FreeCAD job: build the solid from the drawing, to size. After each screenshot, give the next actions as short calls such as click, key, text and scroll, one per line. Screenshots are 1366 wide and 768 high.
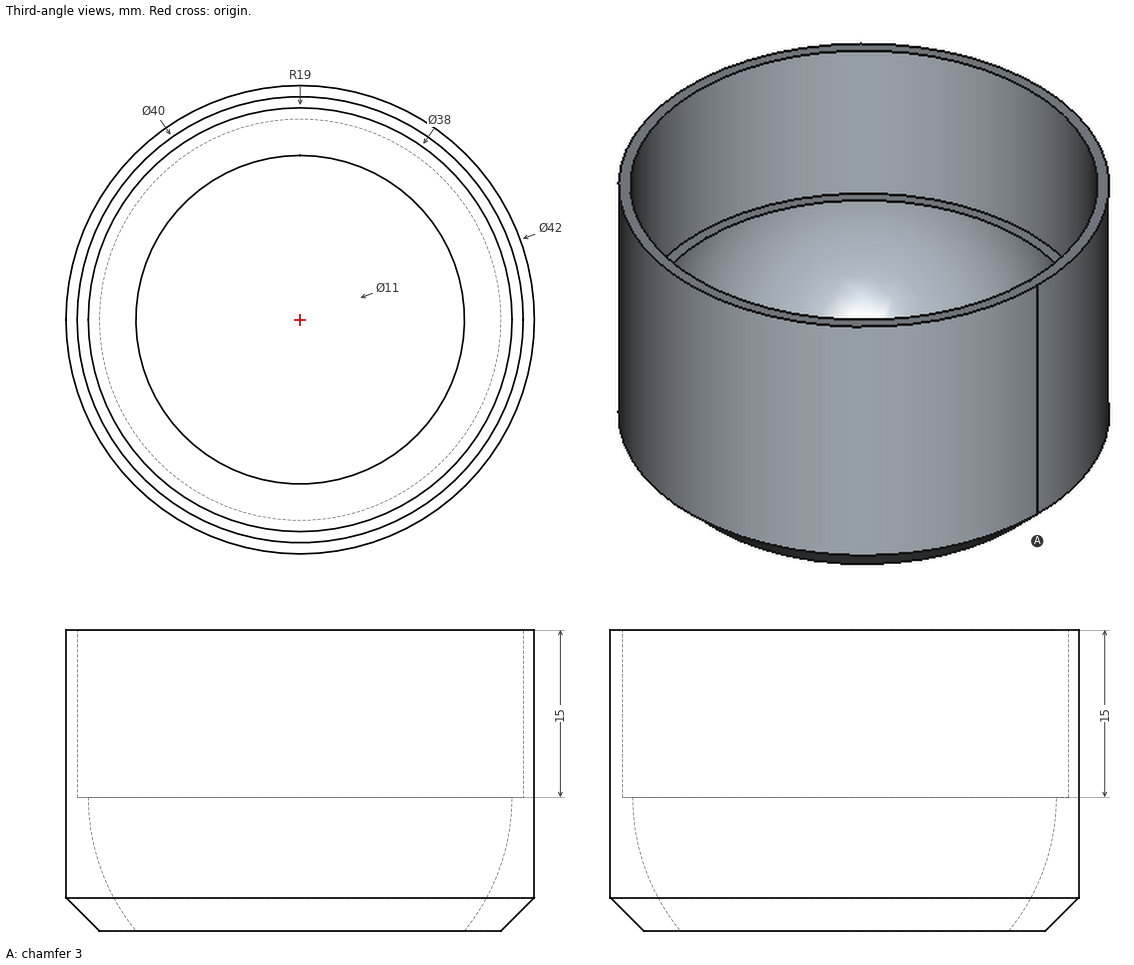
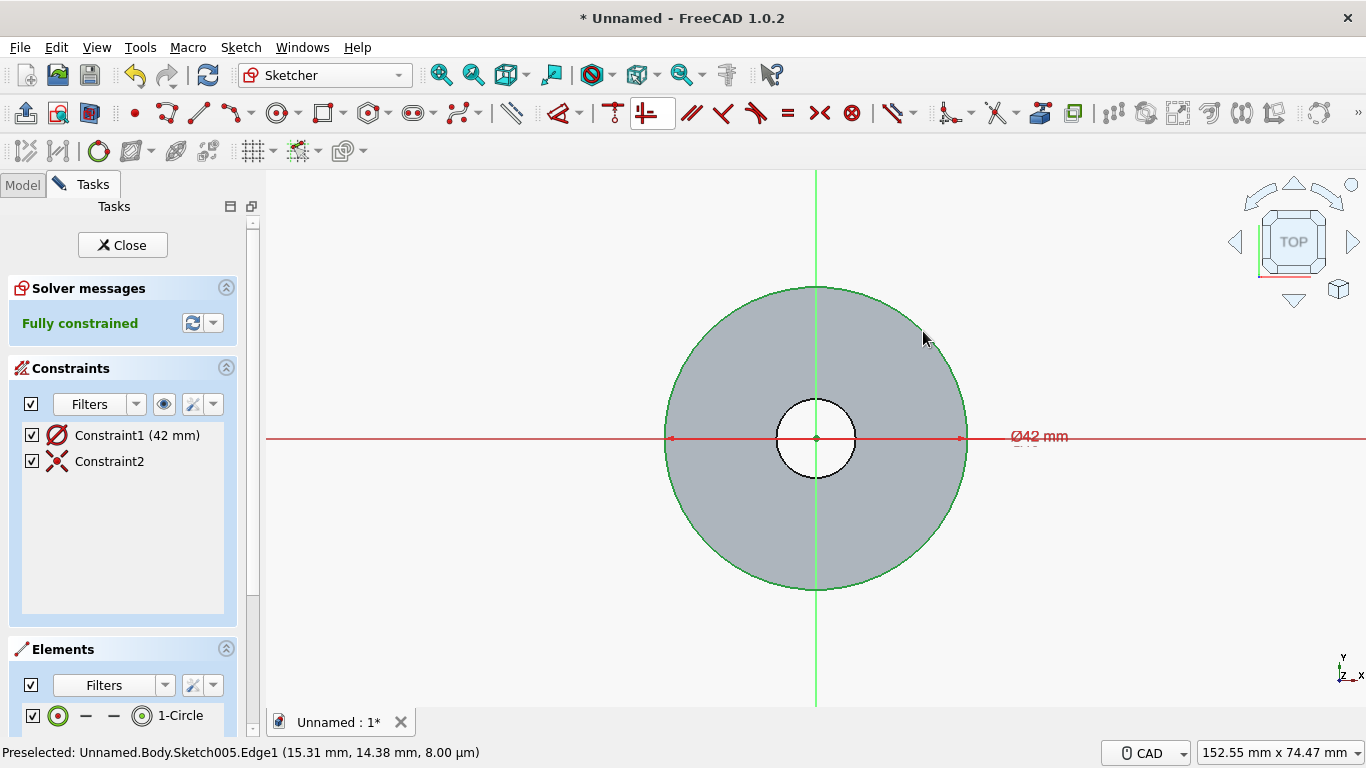
click(123, 245)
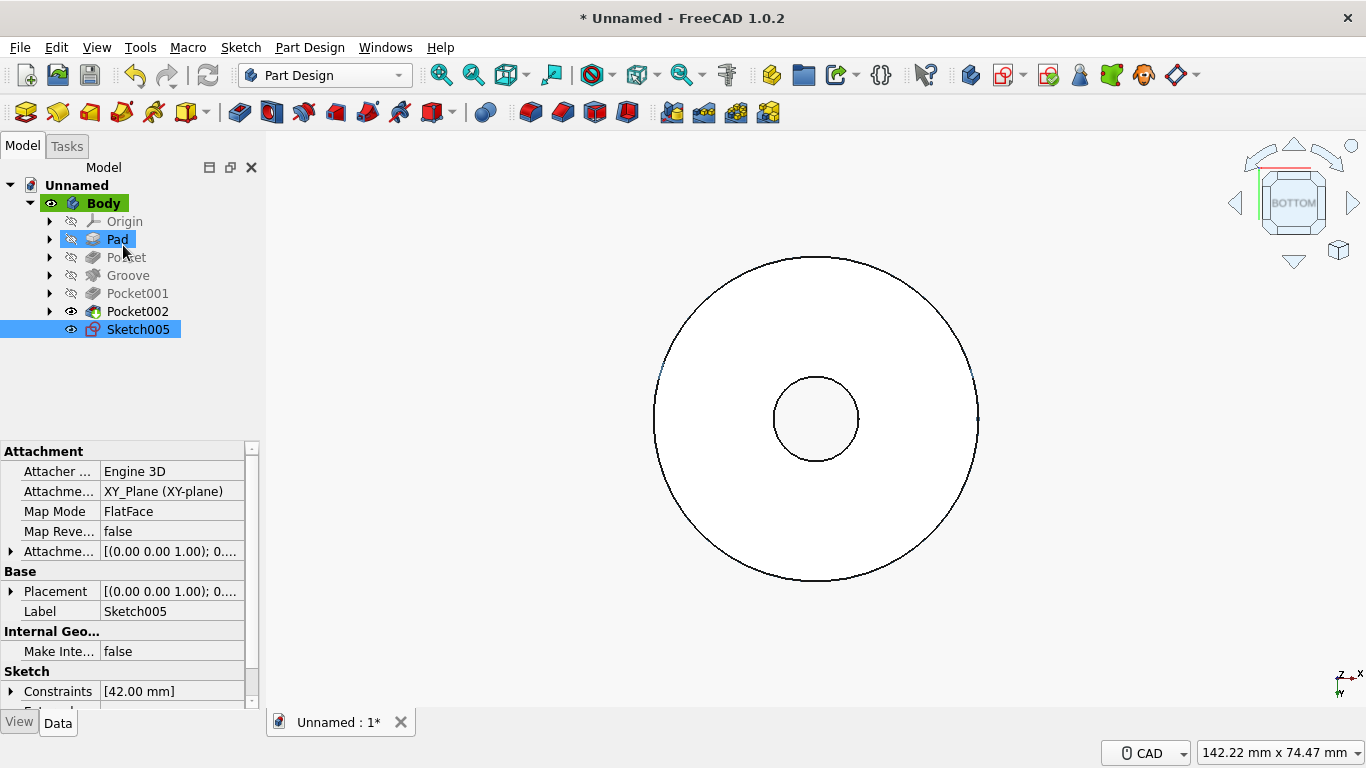
click(240, 112)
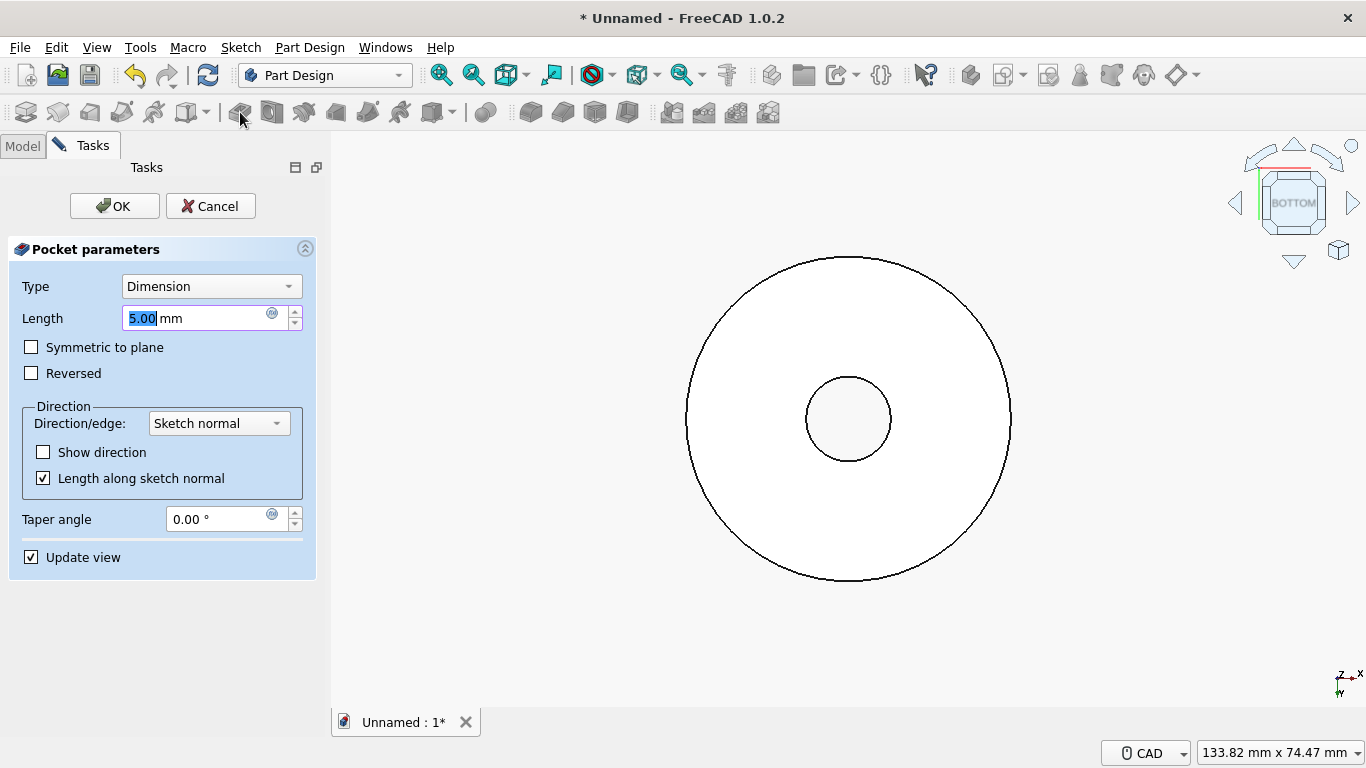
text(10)
key(Tab)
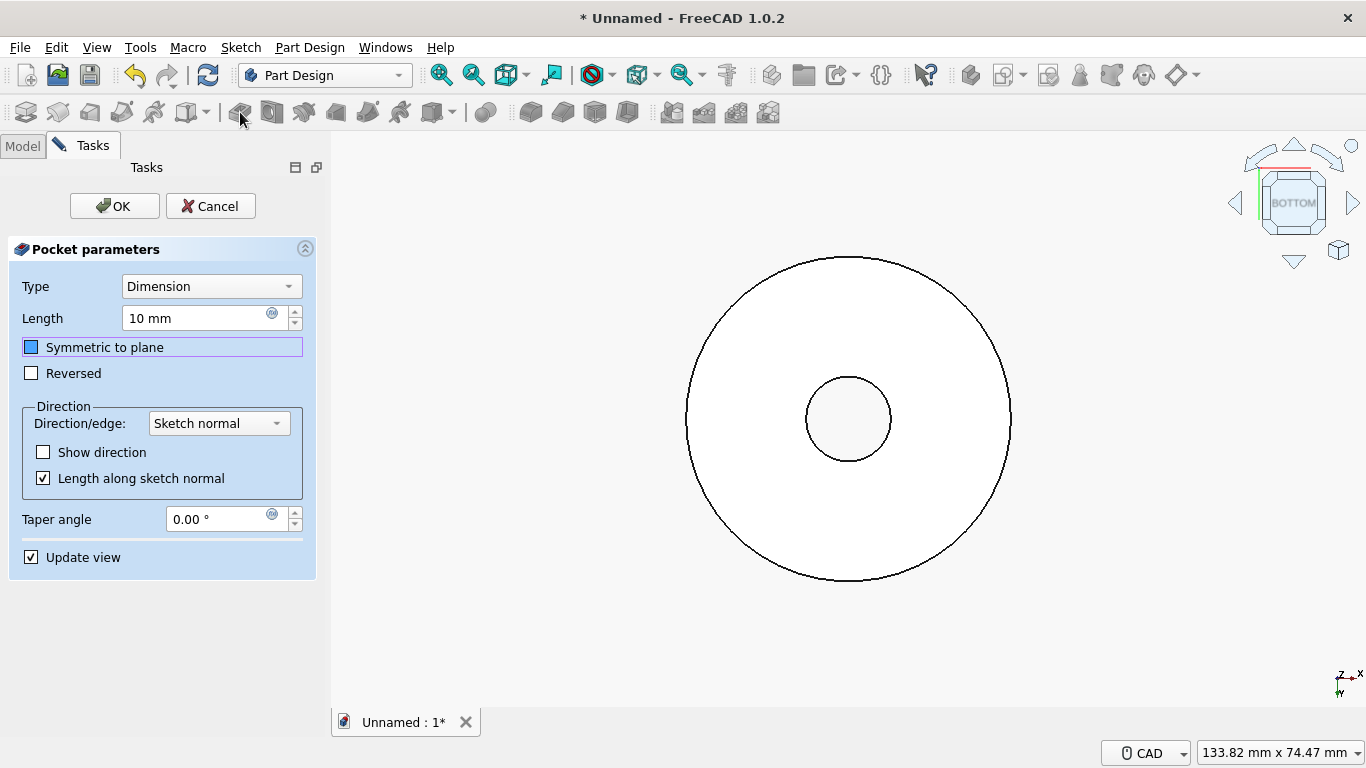
click(30, 373)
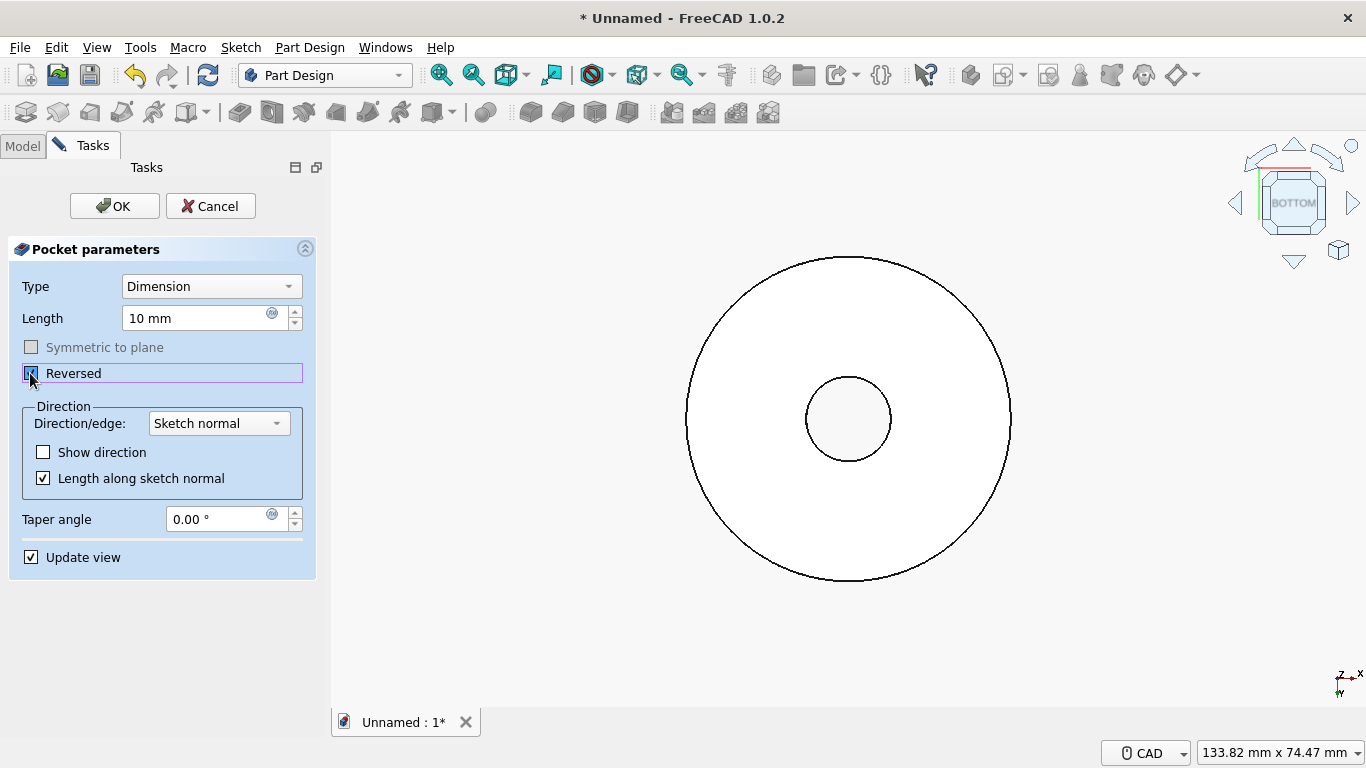
click(115, 206)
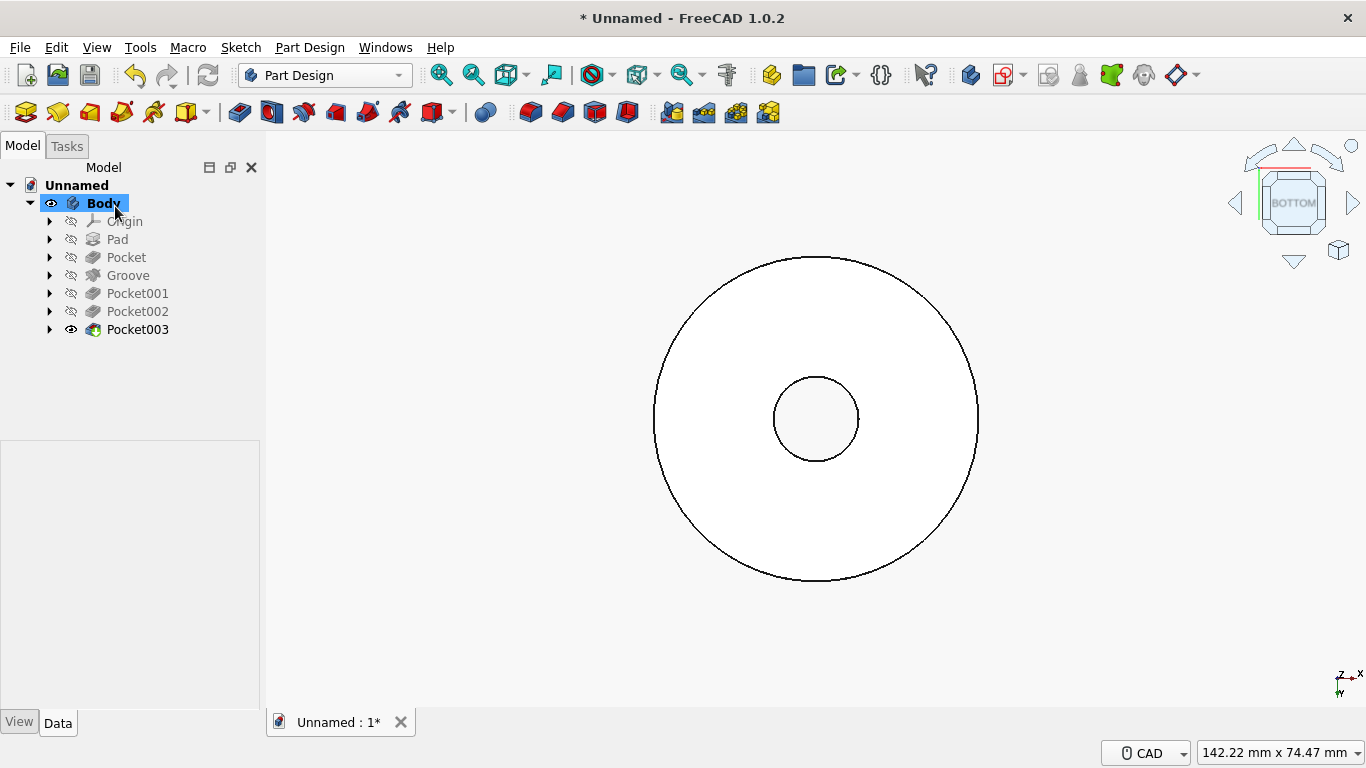
click(909, 372)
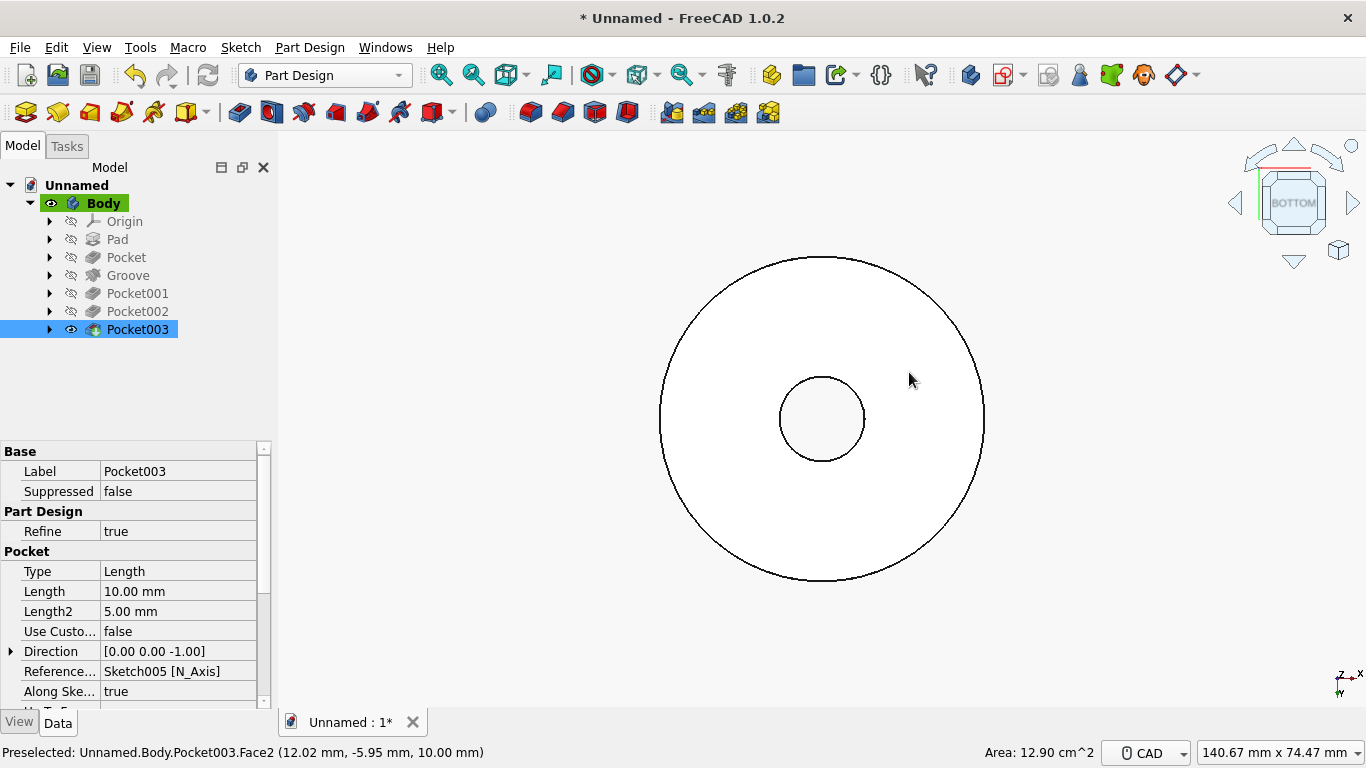
click(1004, 76)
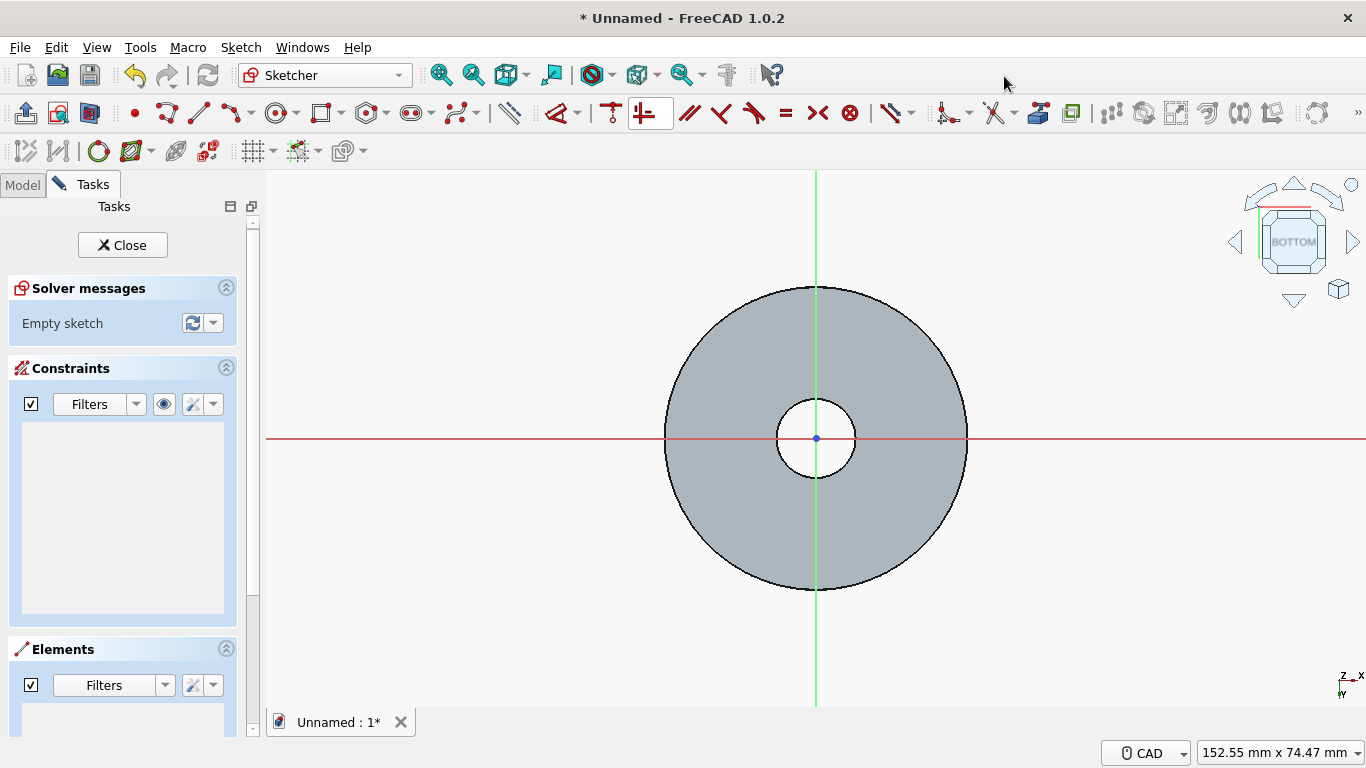
click(276, 114)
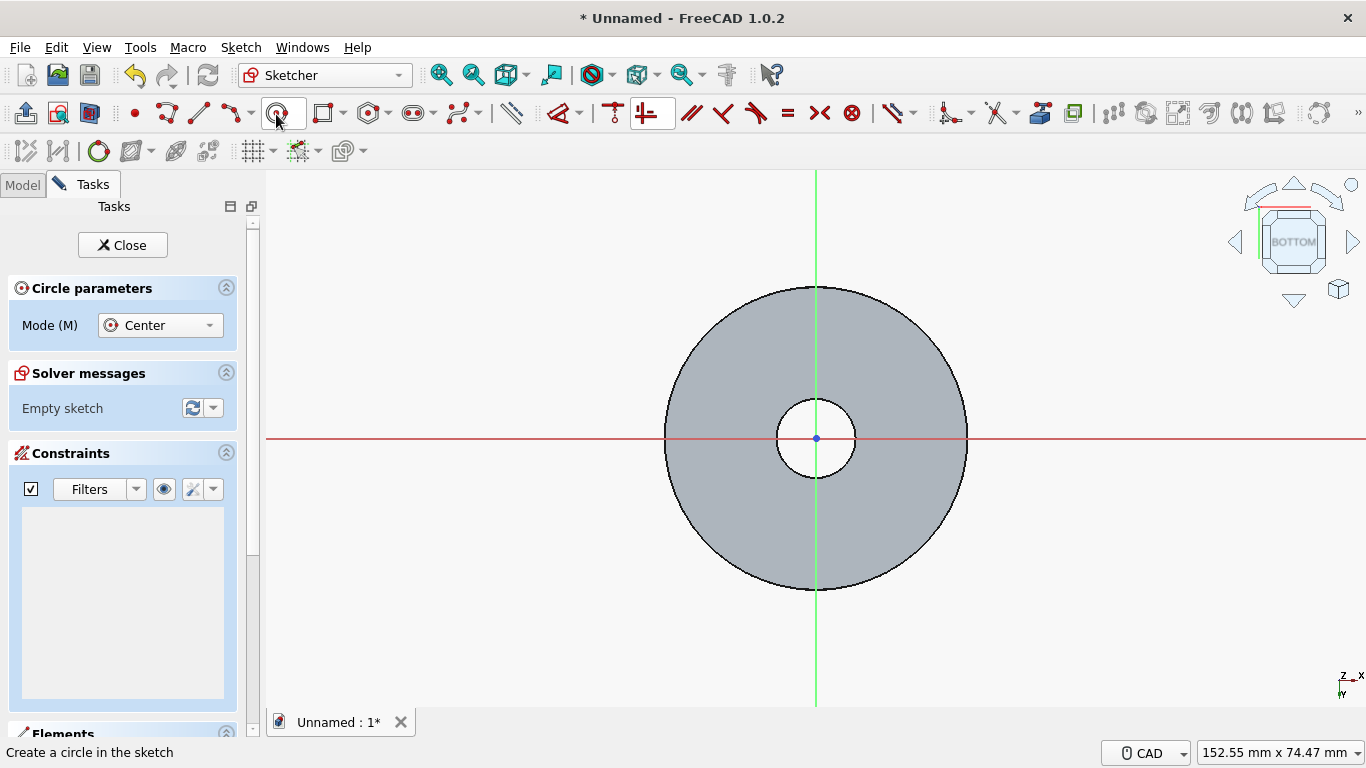
click(816, 439)
move(923, 331)